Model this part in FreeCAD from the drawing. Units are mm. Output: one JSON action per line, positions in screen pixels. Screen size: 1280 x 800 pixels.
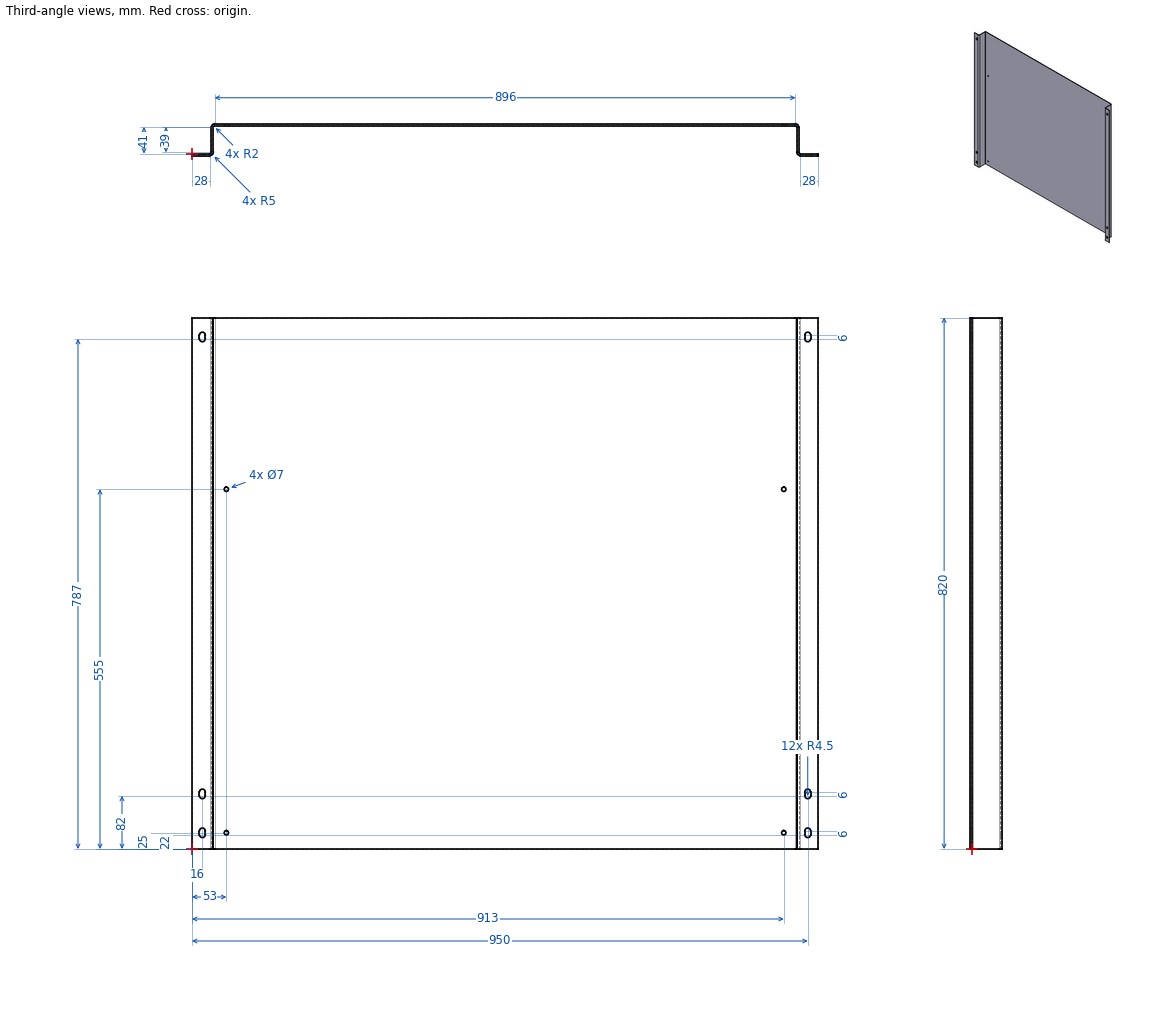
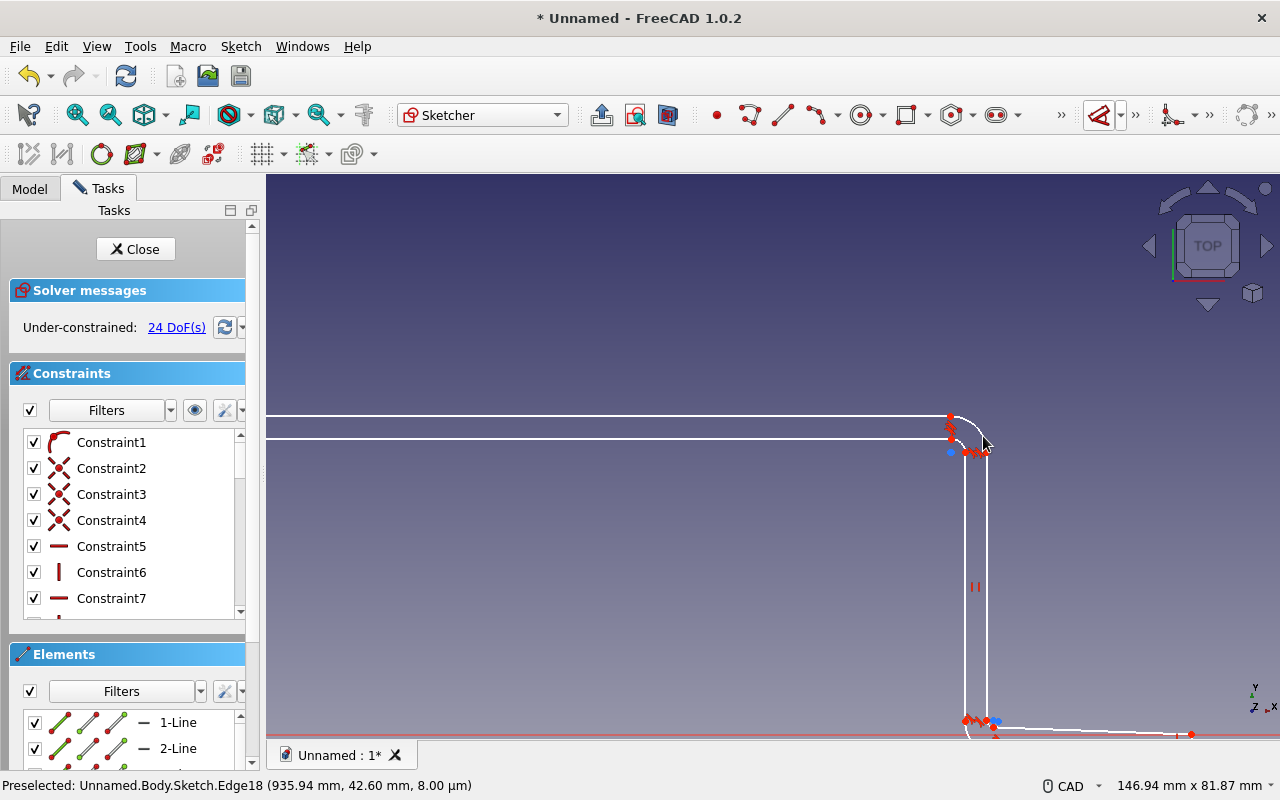
{"action": "scroll", "coordinate": [988, 444], "scroll_direction": "down", "scroll_amount": 12}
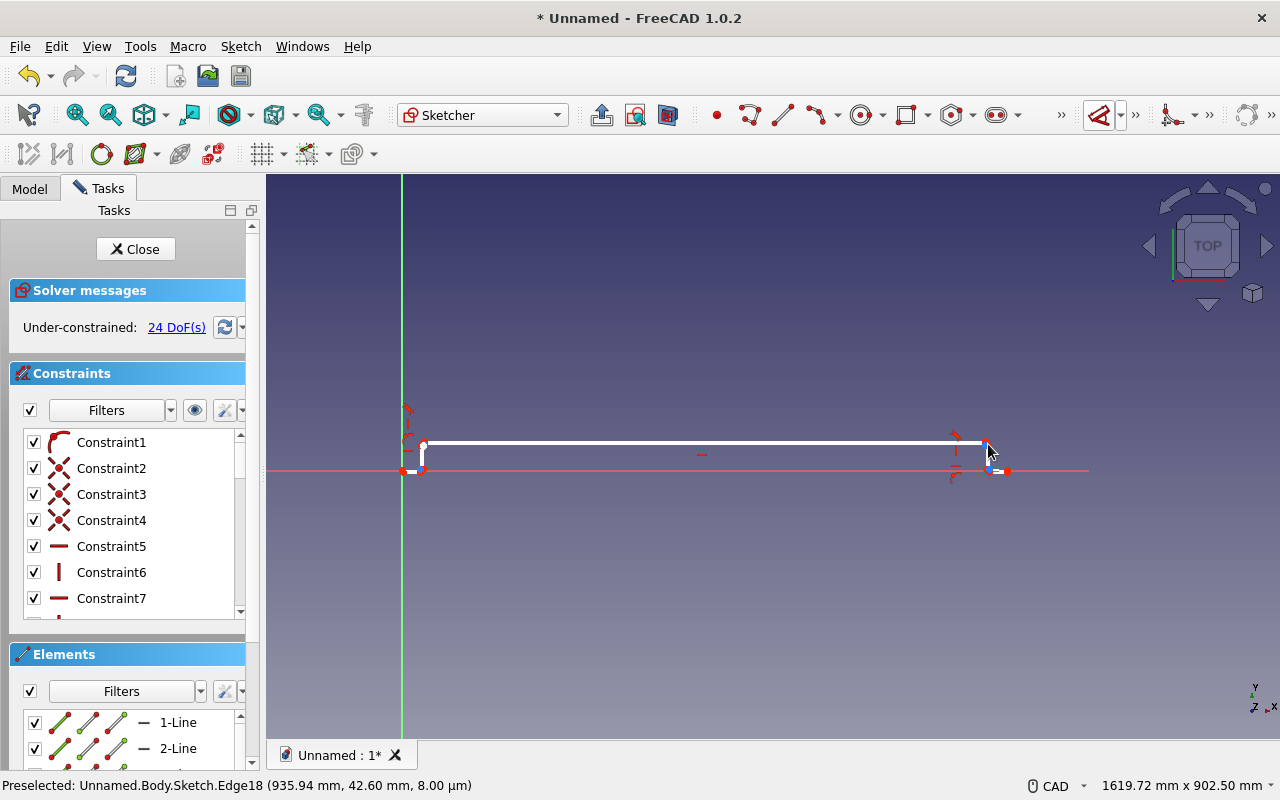
{"action": "scroll", "coordinate": [817, 442], "scroll_direction": "up", "scroll_amount": 10}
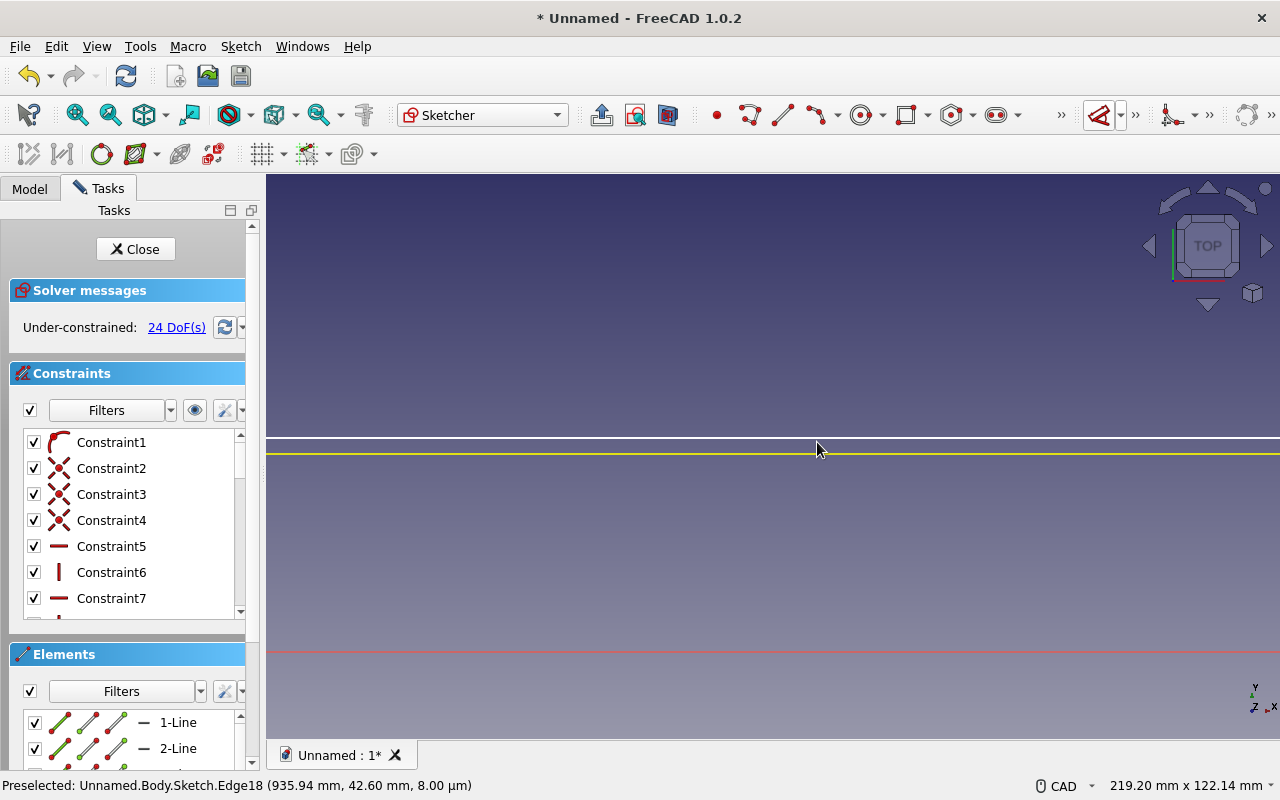
{"action": "left_click", "coordinate": [813, 438]}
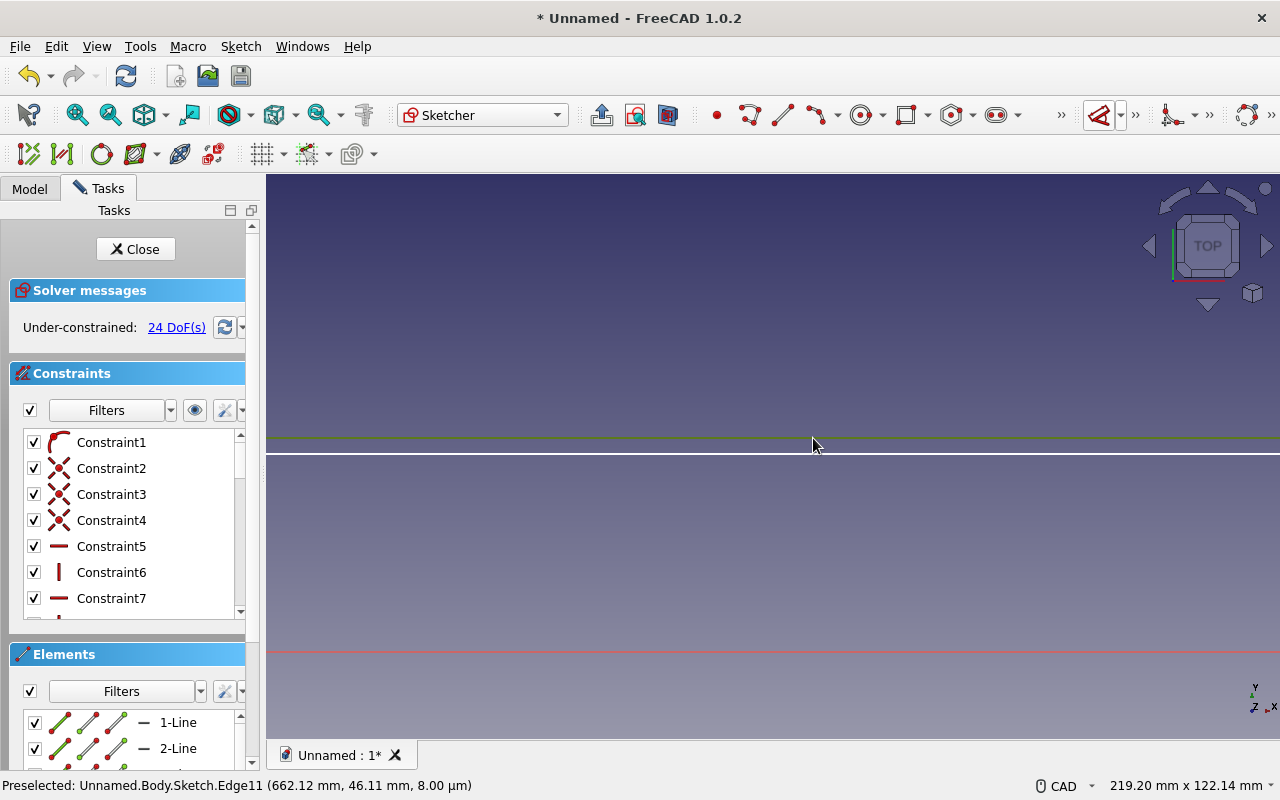
{"action": "scroll", "coordinate": [817, 442], "scroll_direction": "down", "scroll_amount": 10}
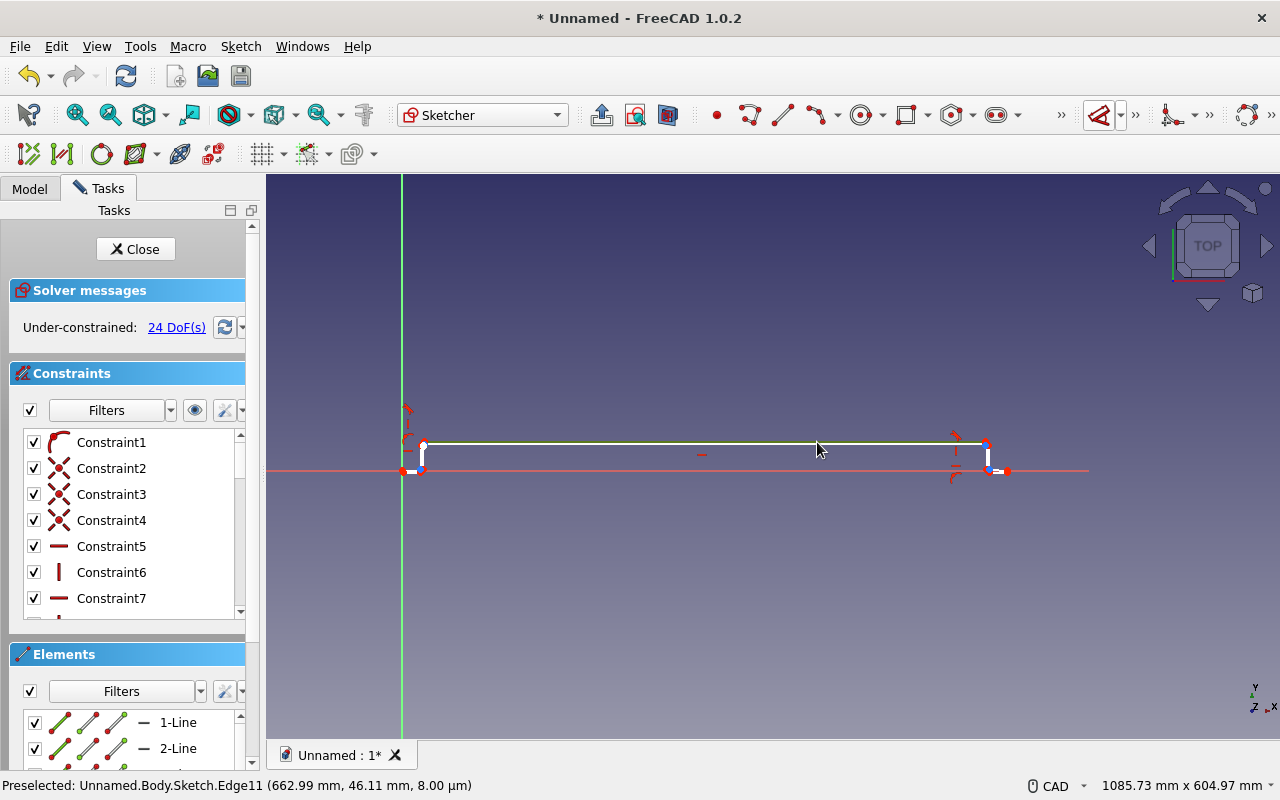
{"action": "scroll", "coordinate": [423, 442], "scroll_direction": "up", "scroll_amount": 12}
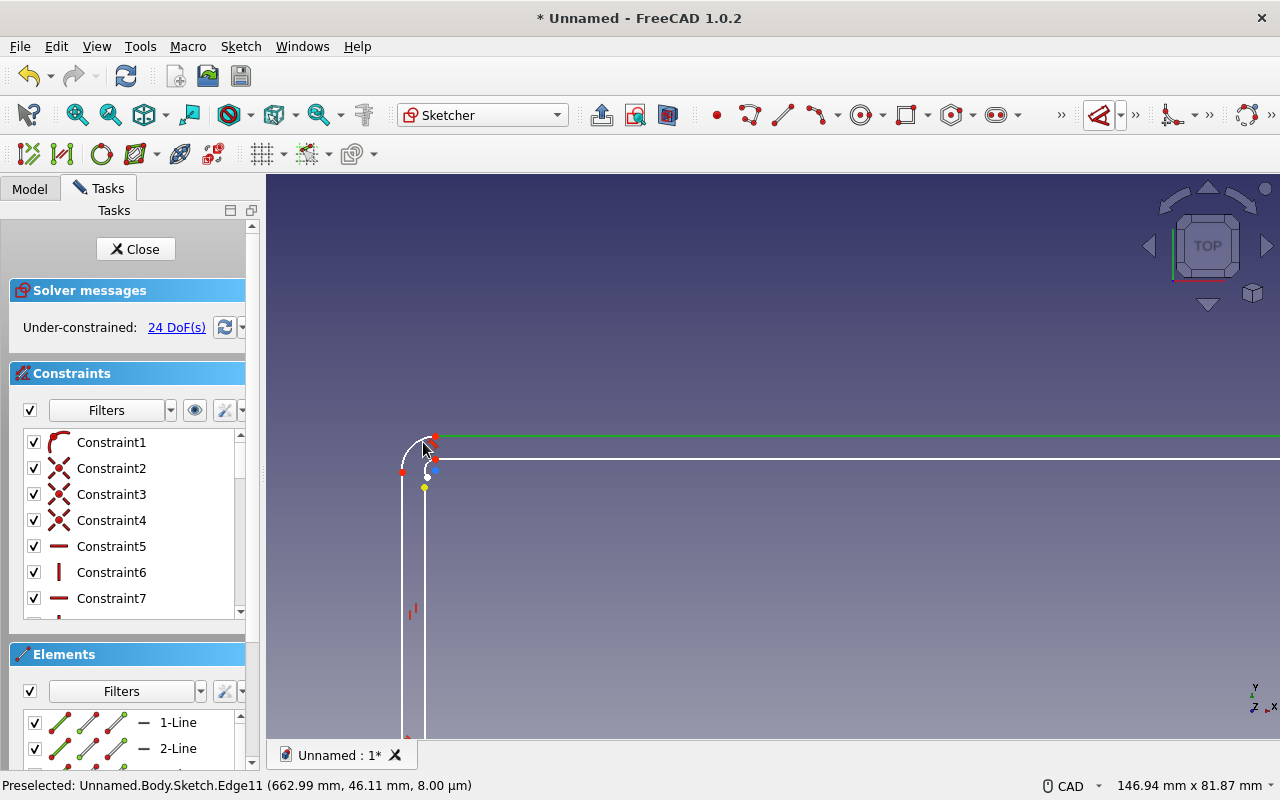
{"action": "left_click", "coordinate": [420, 440]}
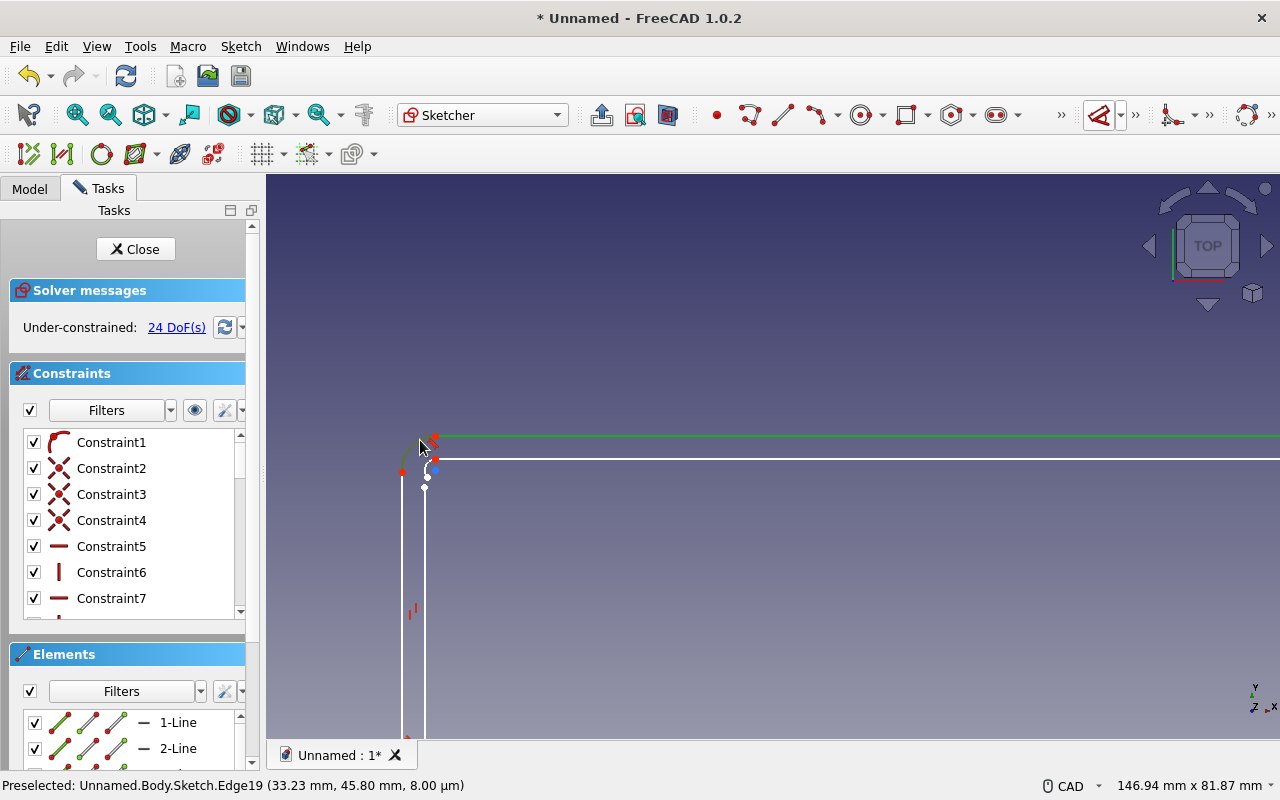
{"action": "key", "text": "t"}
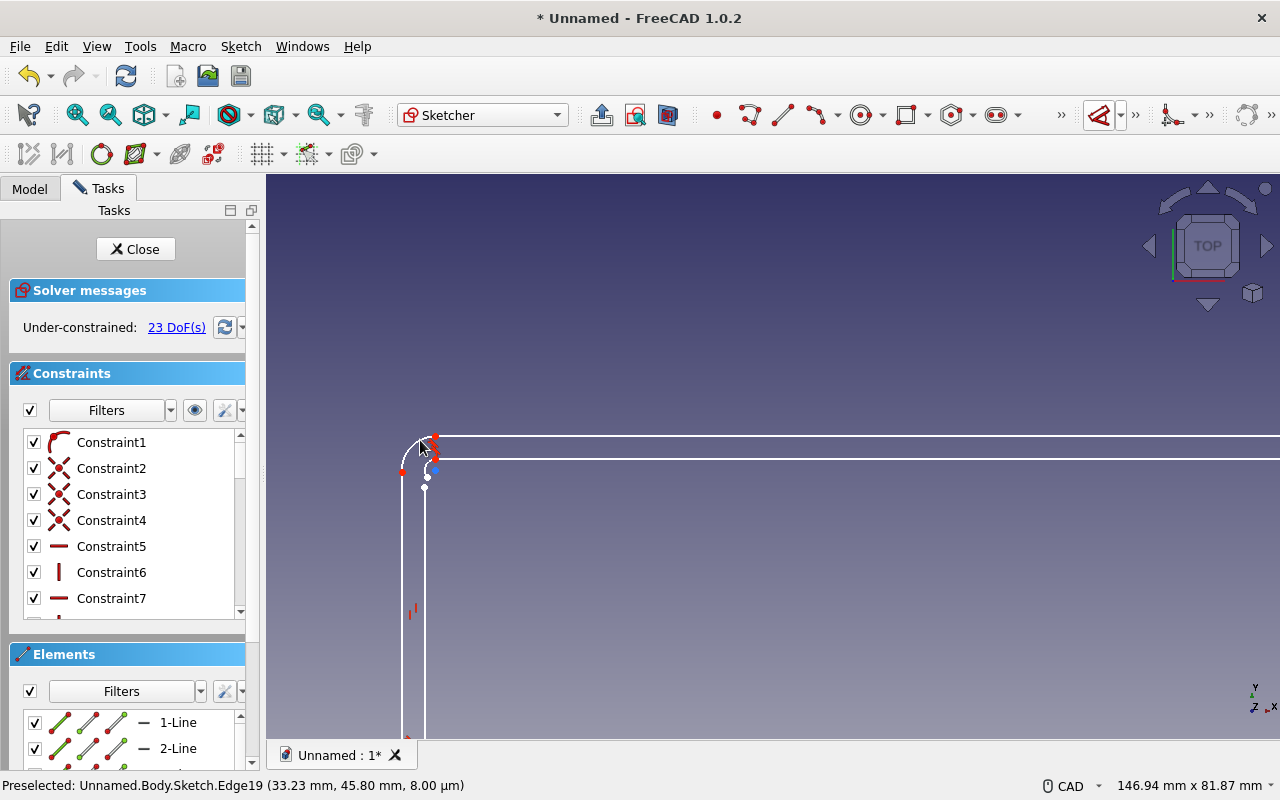
{"action": "left_click", "coordinate": [402, 553]}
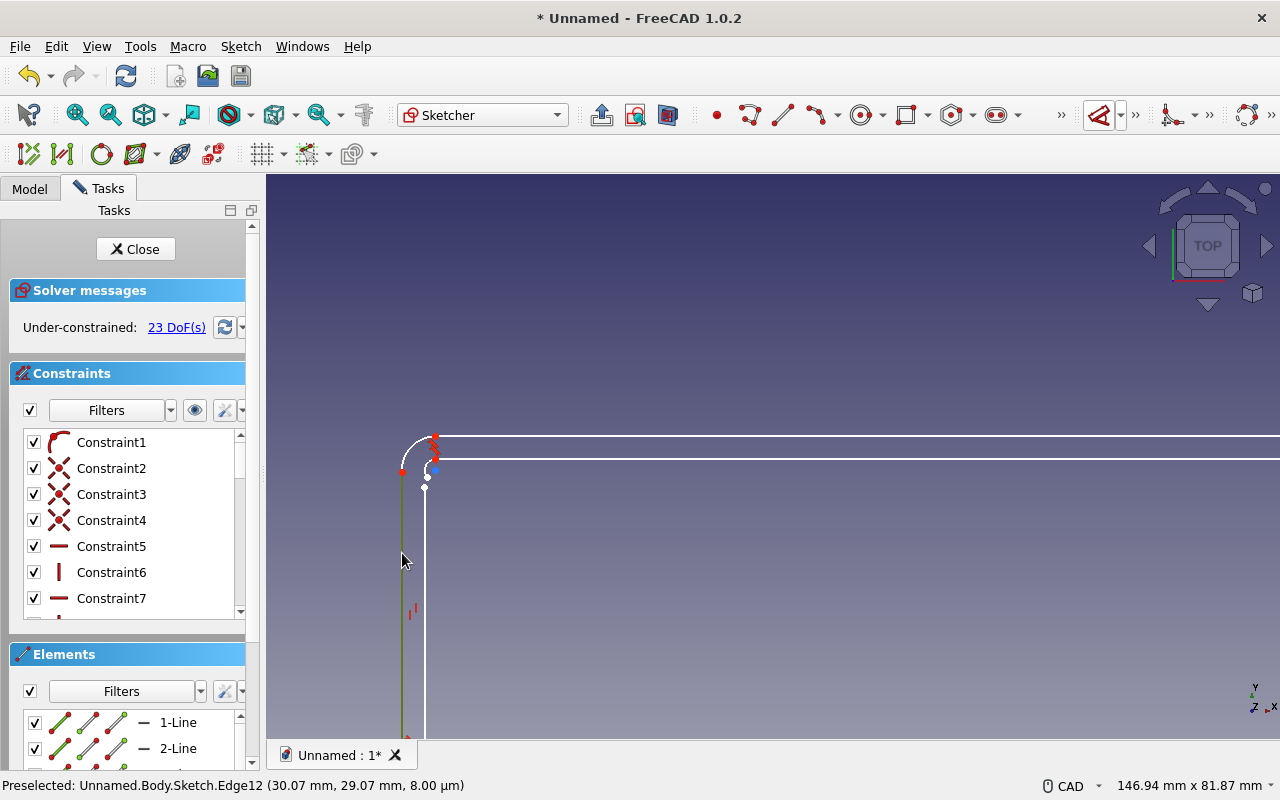
{"action": "left_click", "coordinate": [420, 440]}